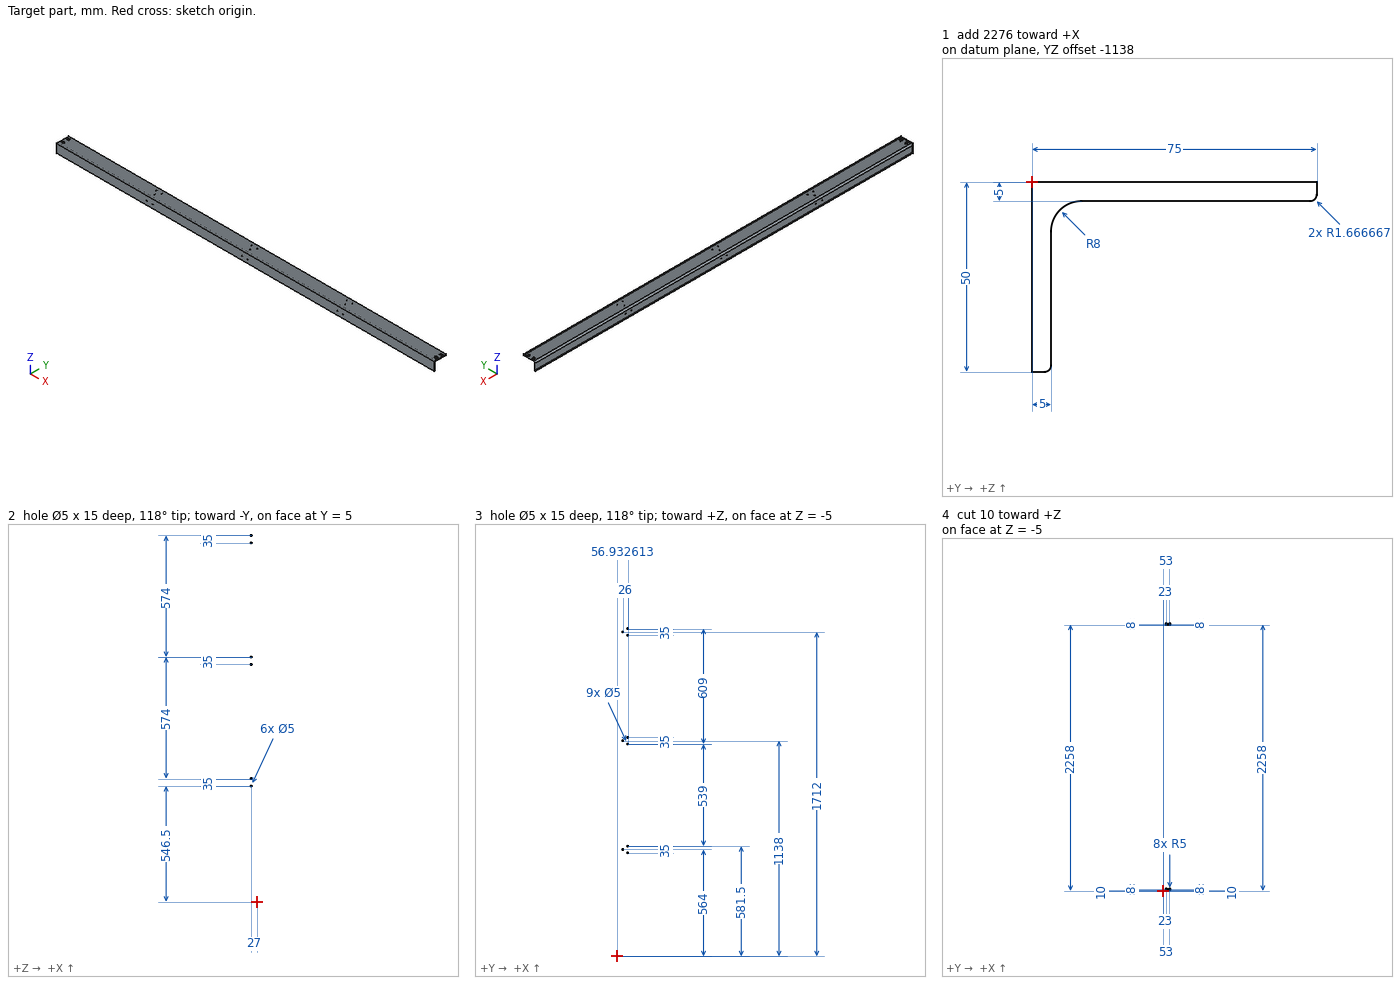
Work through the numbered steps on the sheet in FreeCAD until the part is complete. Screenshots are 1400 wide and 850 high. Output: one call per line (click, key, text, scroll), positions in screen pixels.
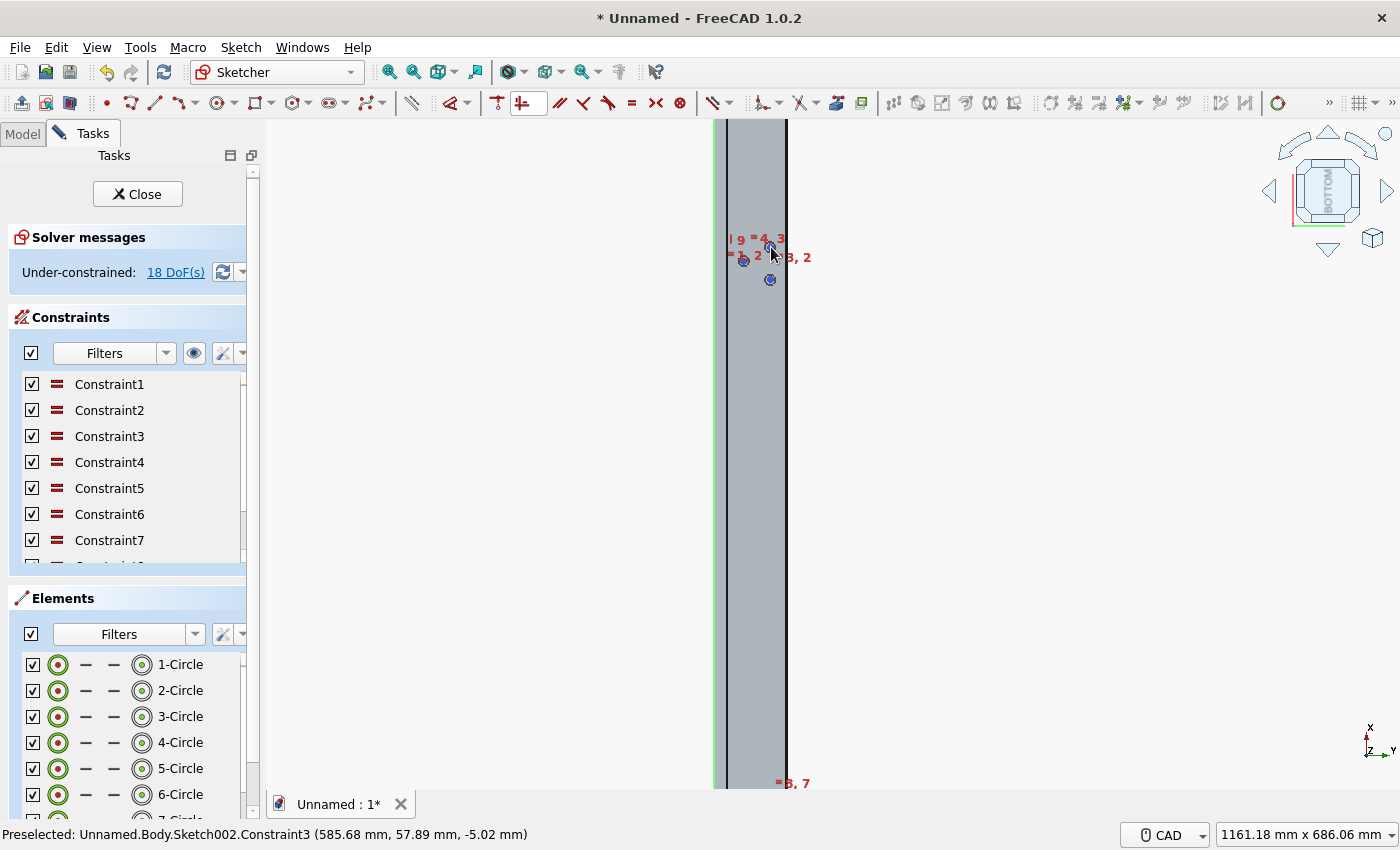
click(770, 247)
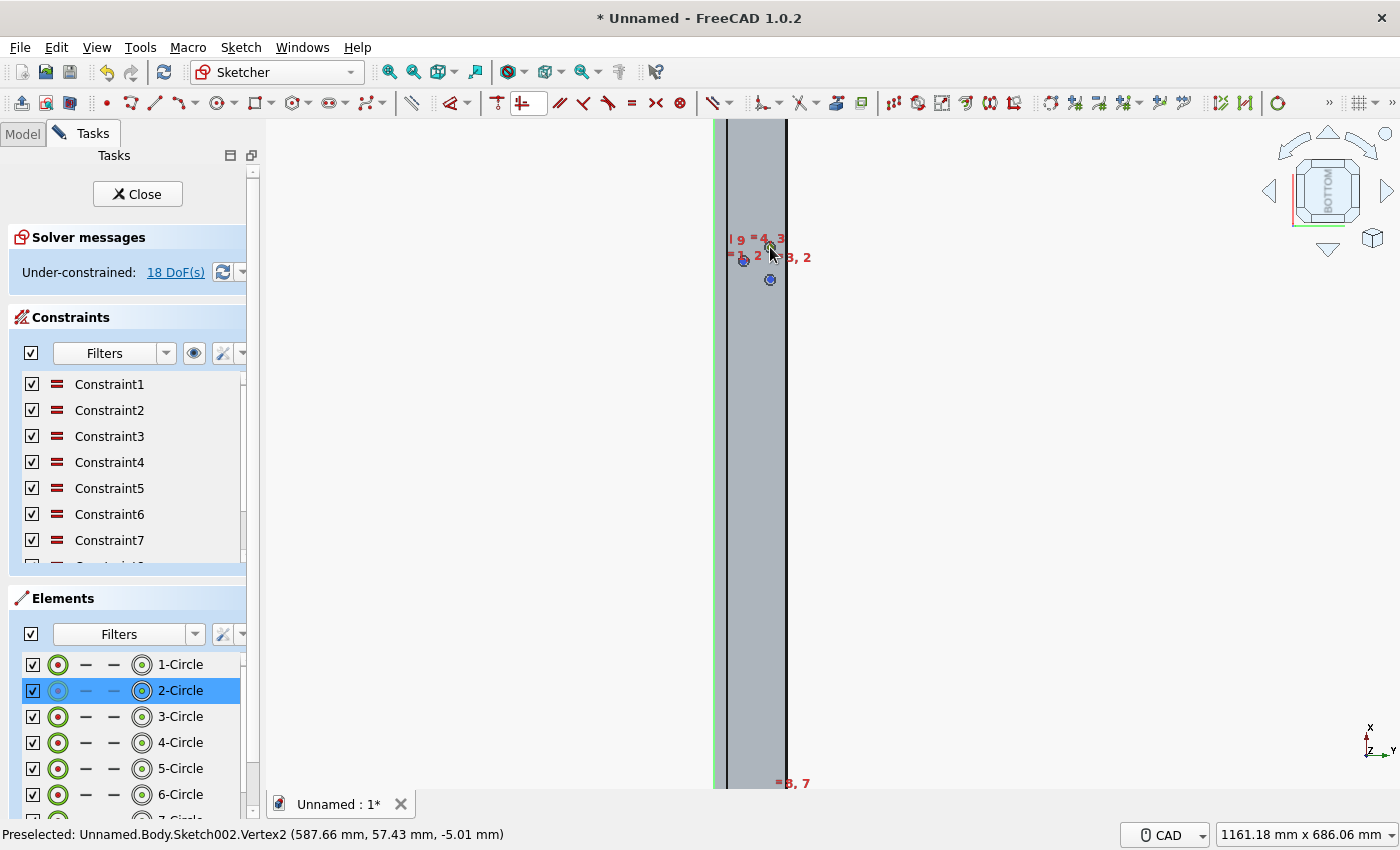
click(770, 280)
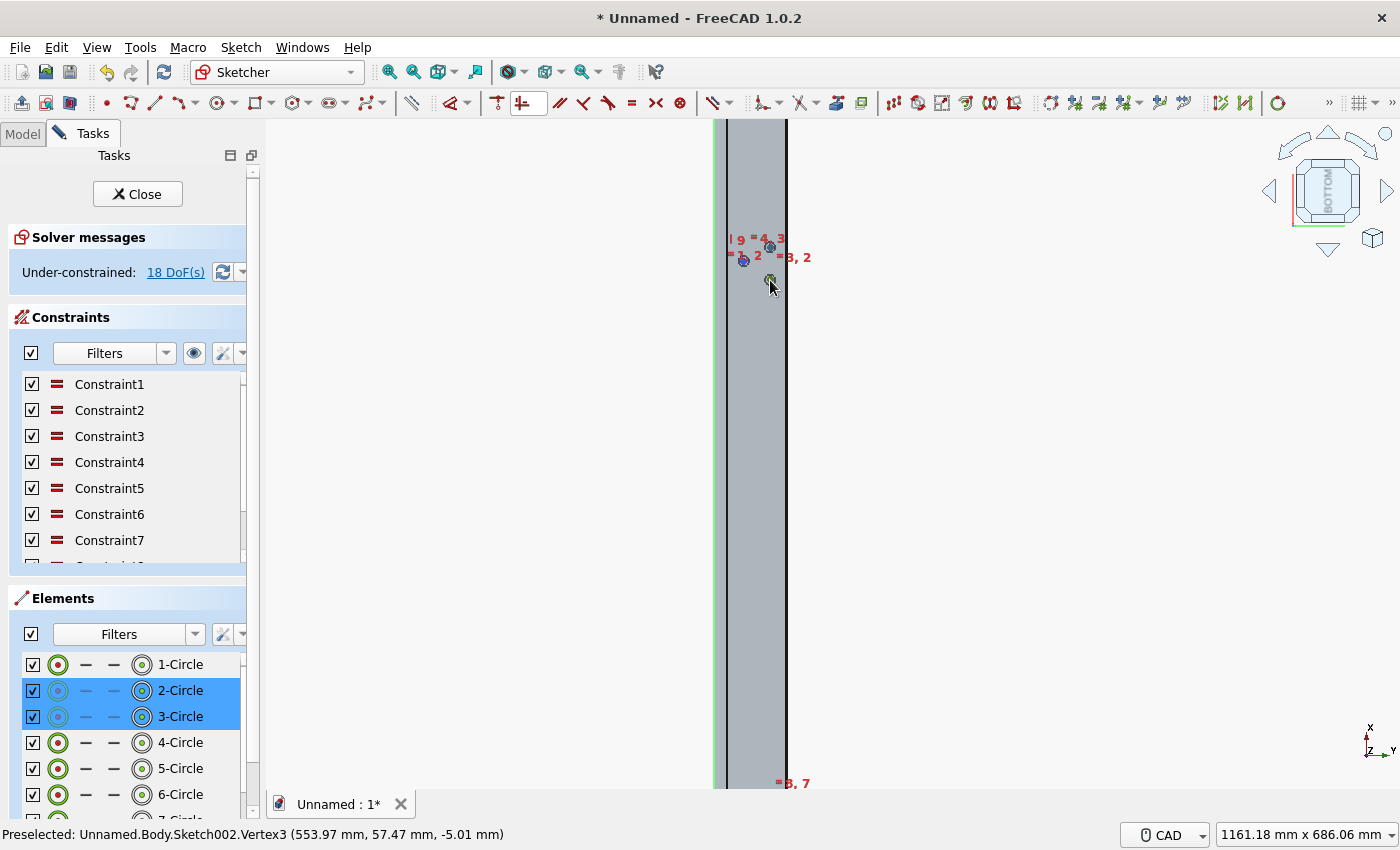
key(v)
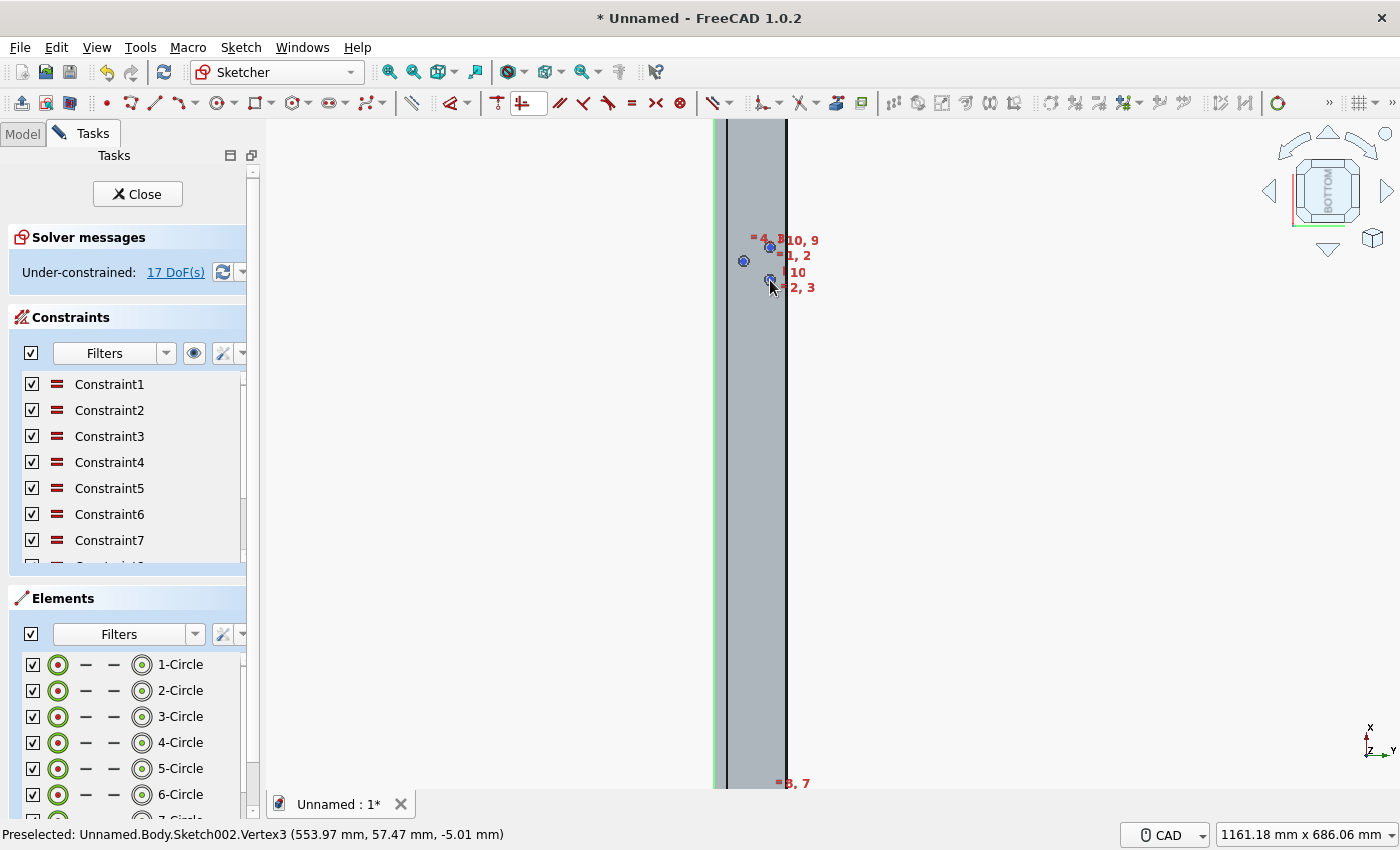
scroll(772, 247, down, 7)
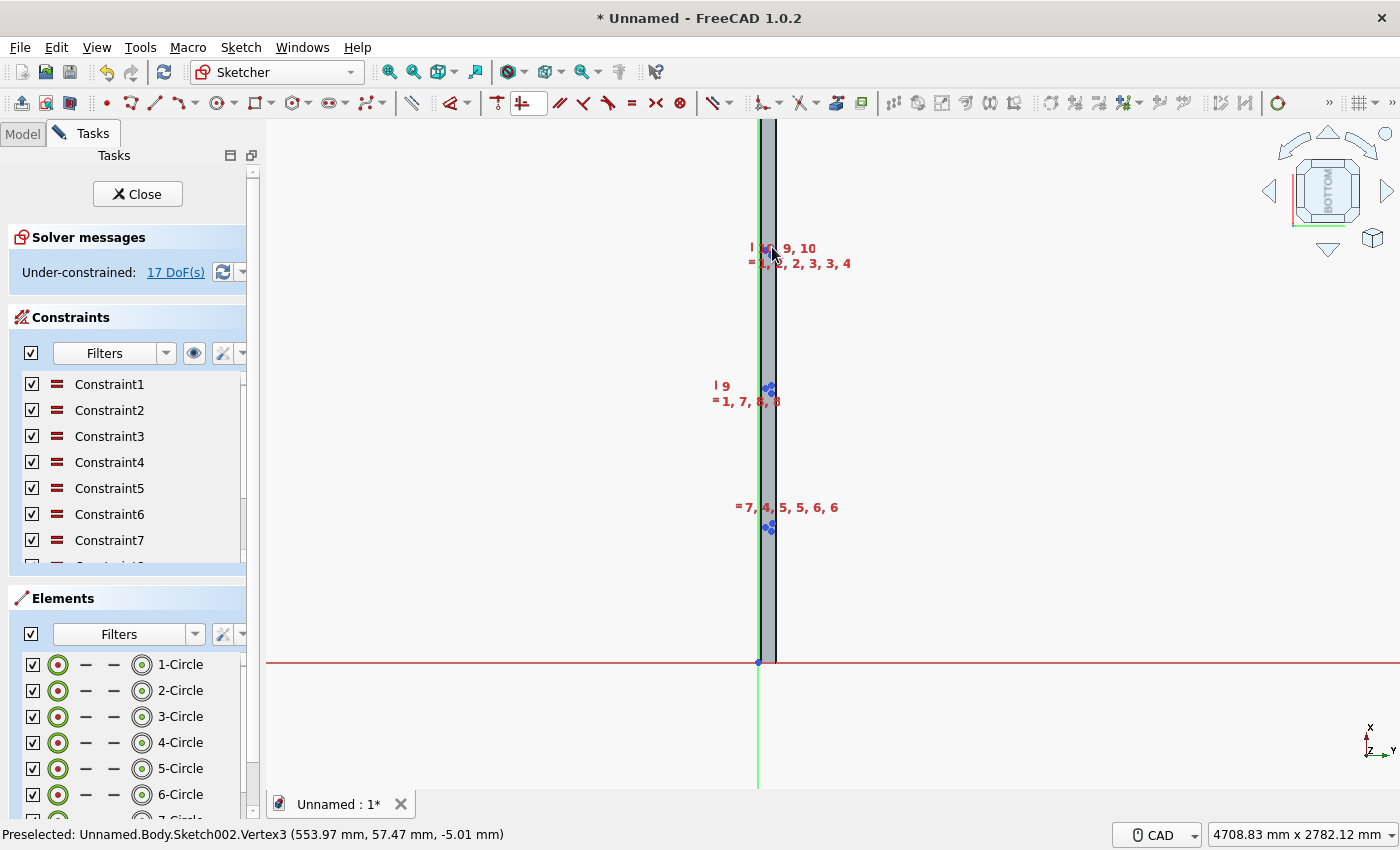
scroll(772, 394, up, 3)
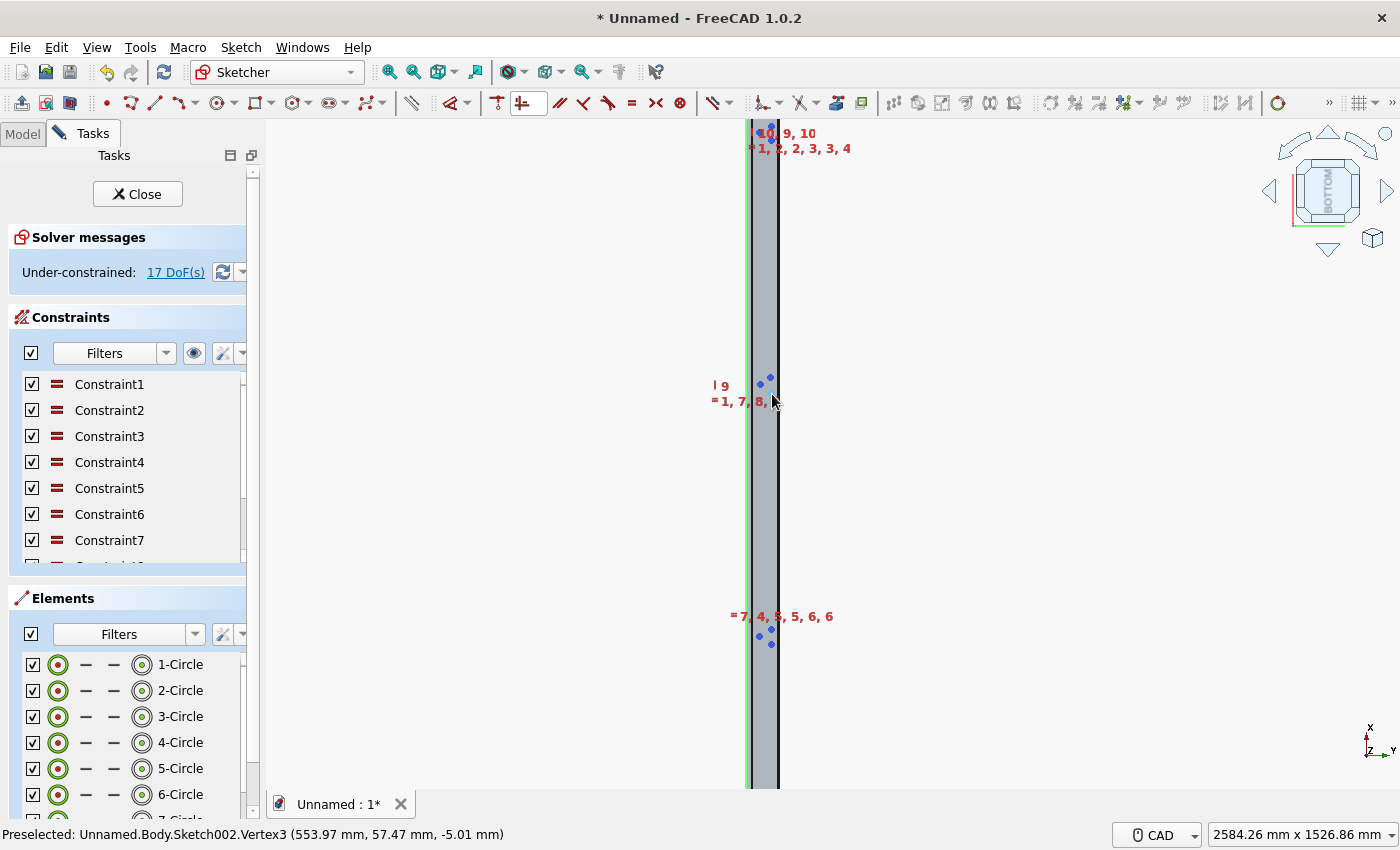
click(771, 393)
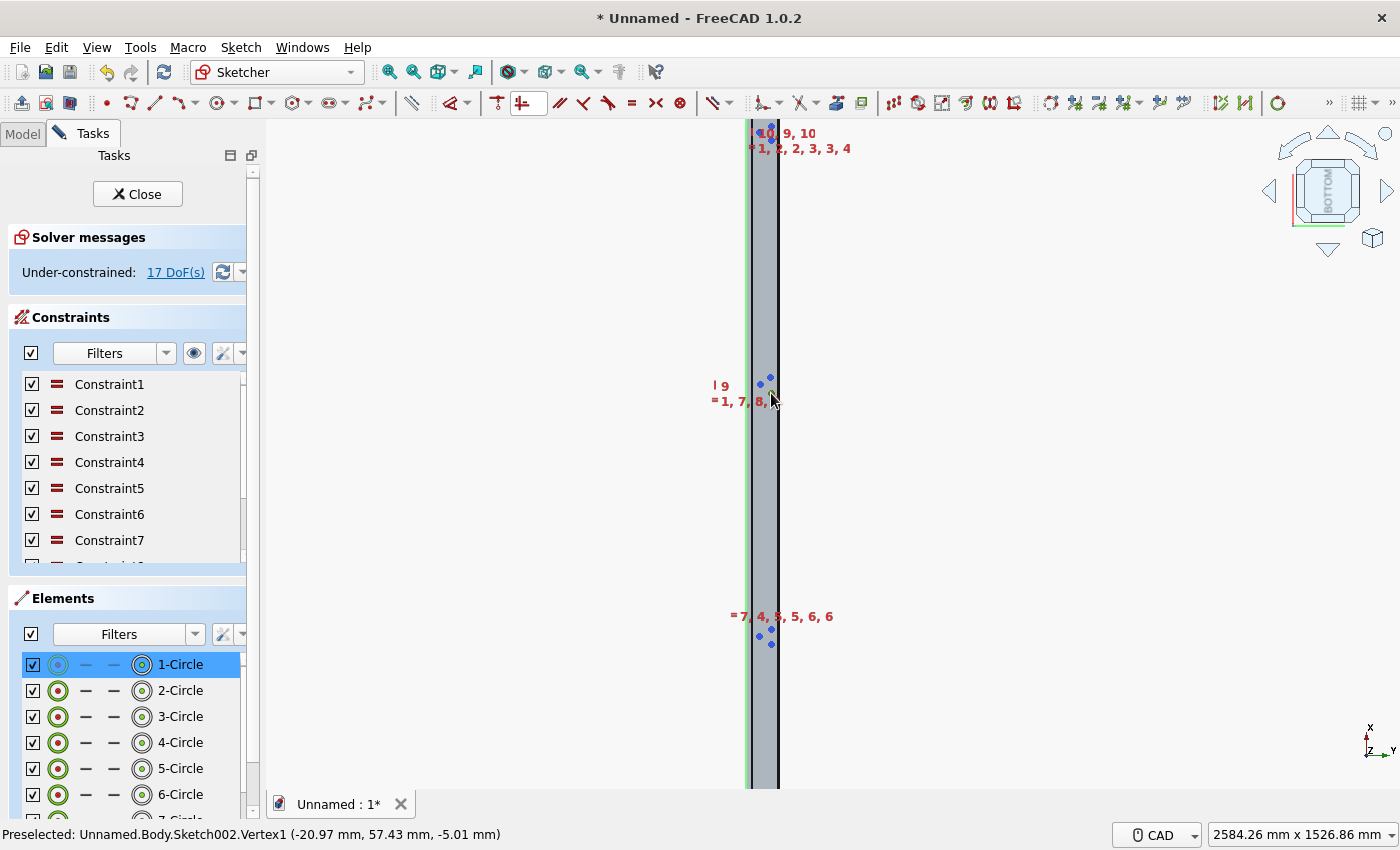
click(772, 629)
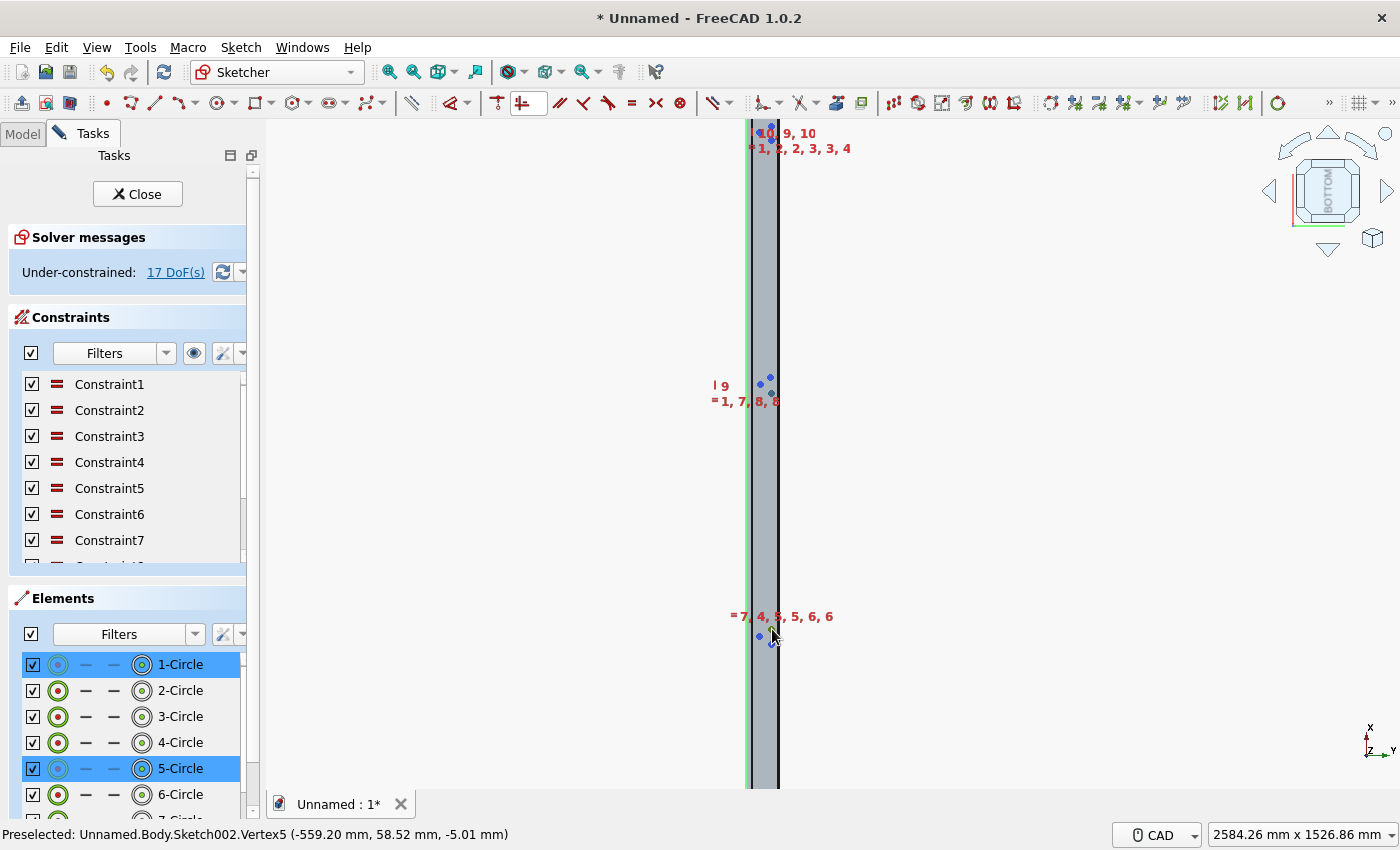
click(542, 104)